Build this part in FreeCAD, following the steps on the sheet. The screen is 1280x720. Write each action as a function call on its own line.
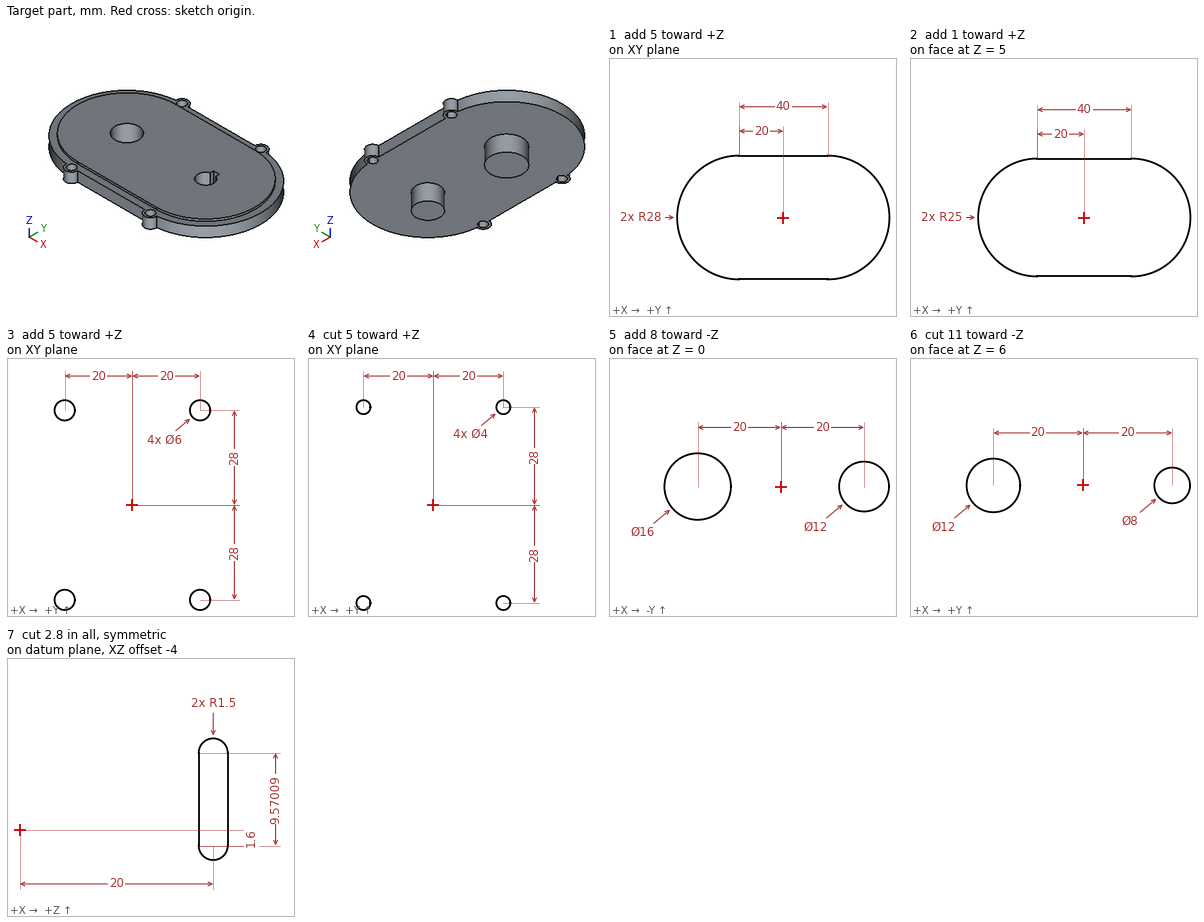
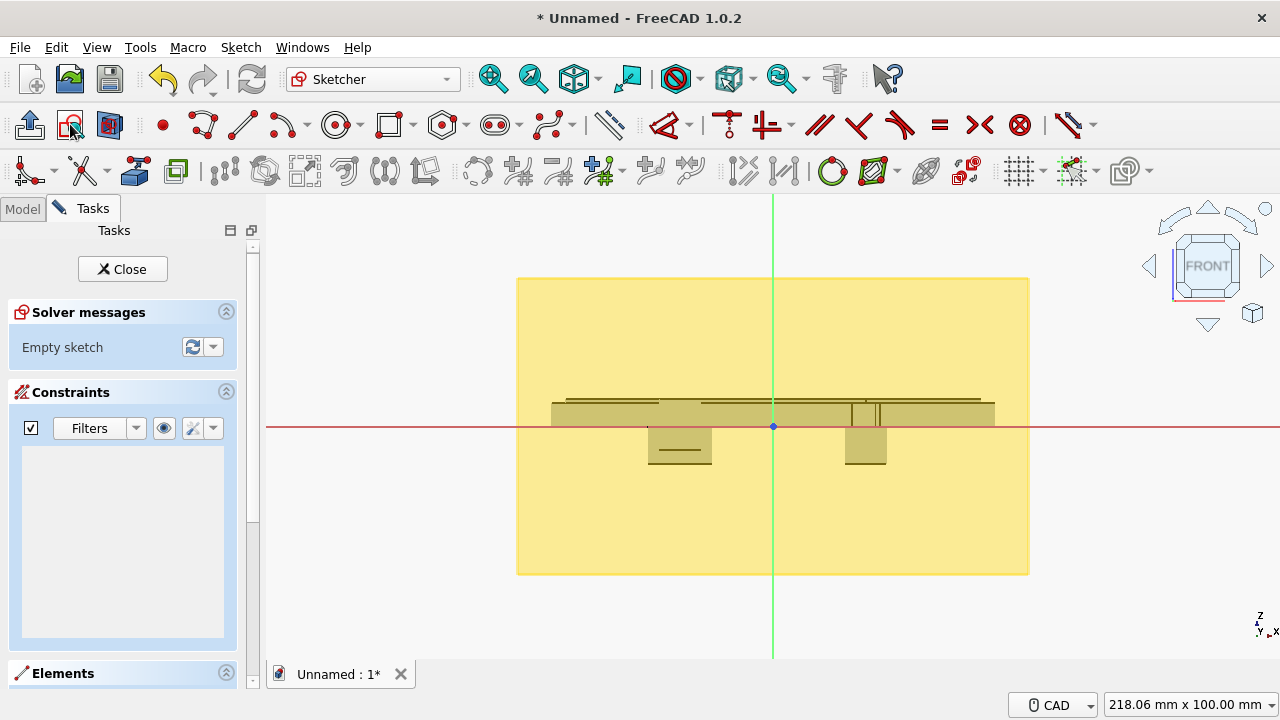
scroll(853, 408, up, 8)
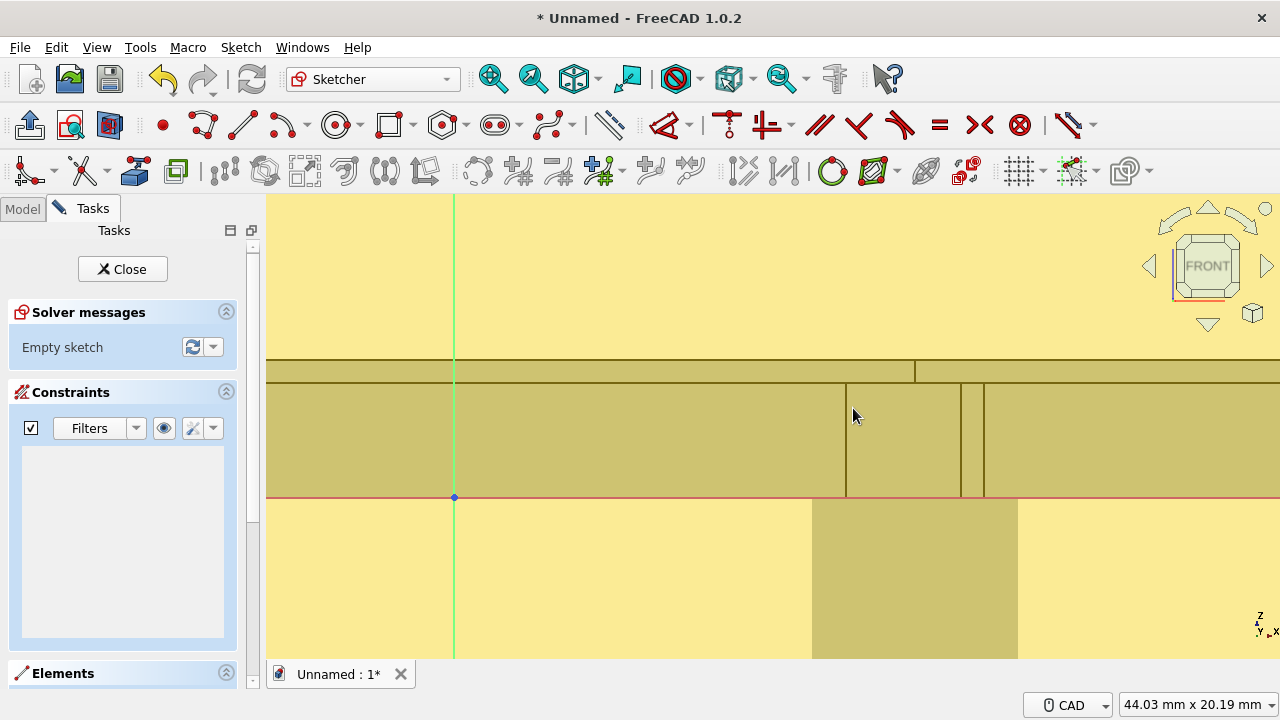
click(496, 126)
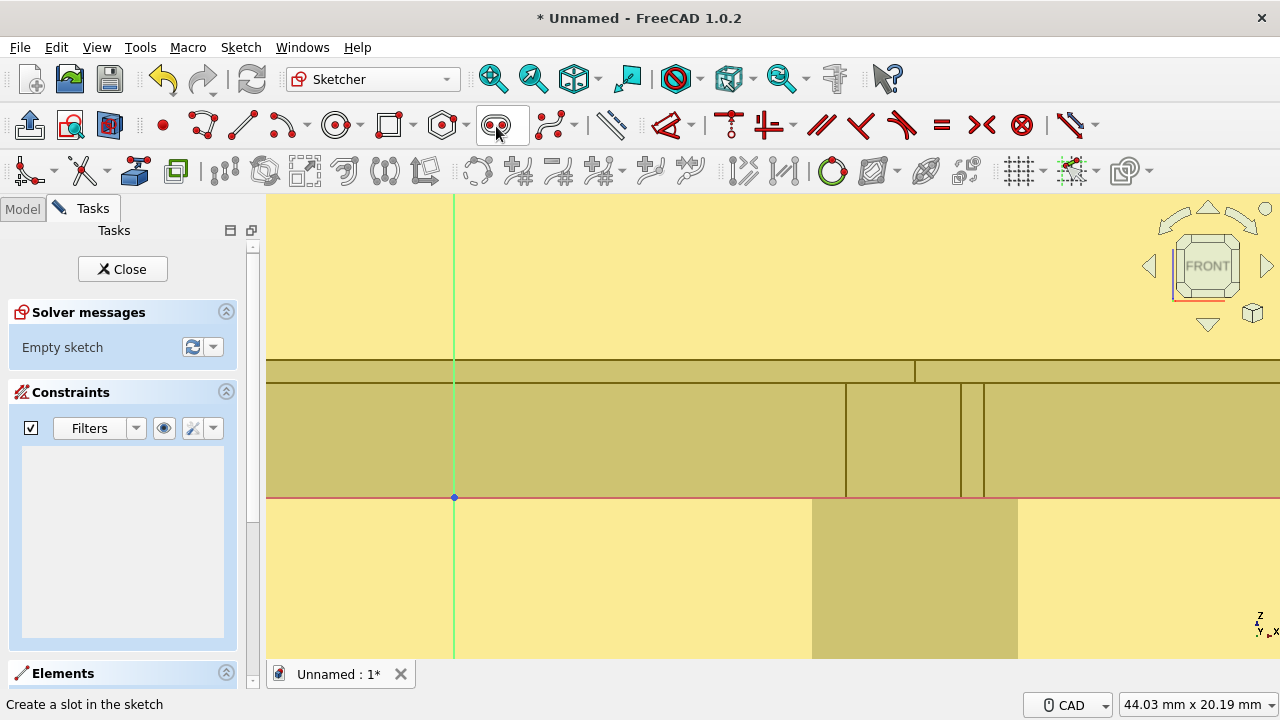
click(915, 535)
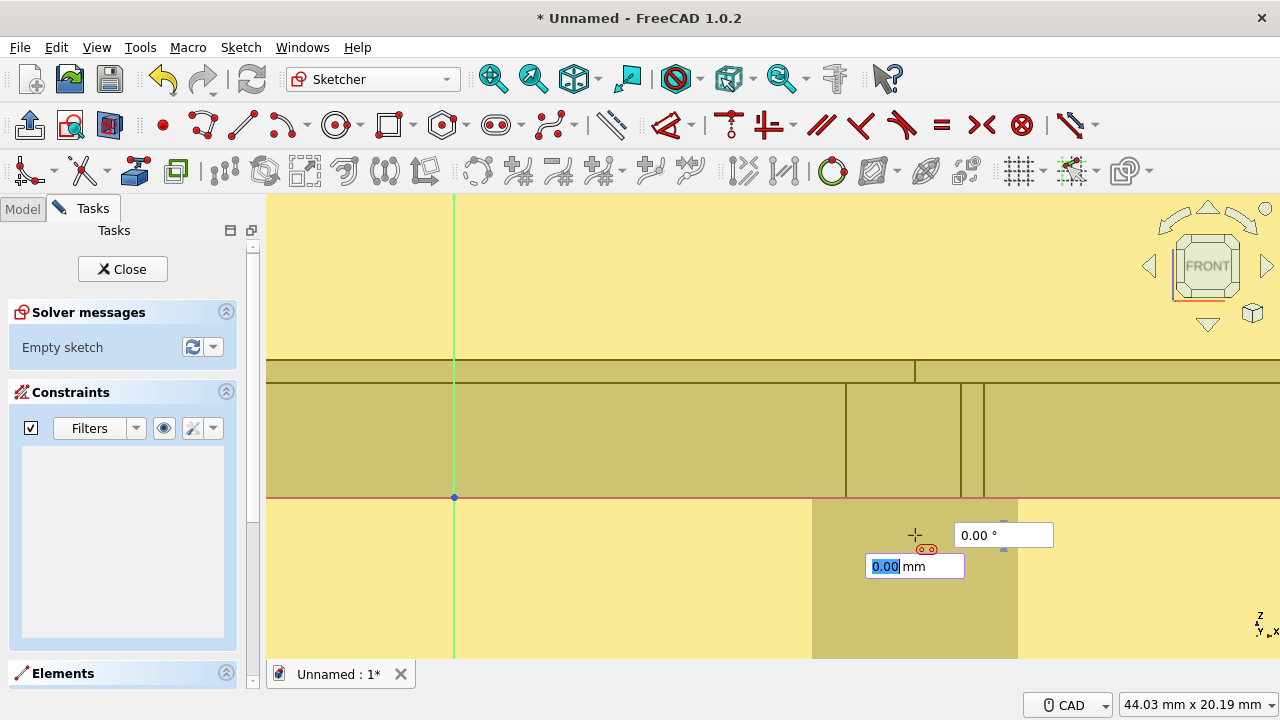
click(915, 314)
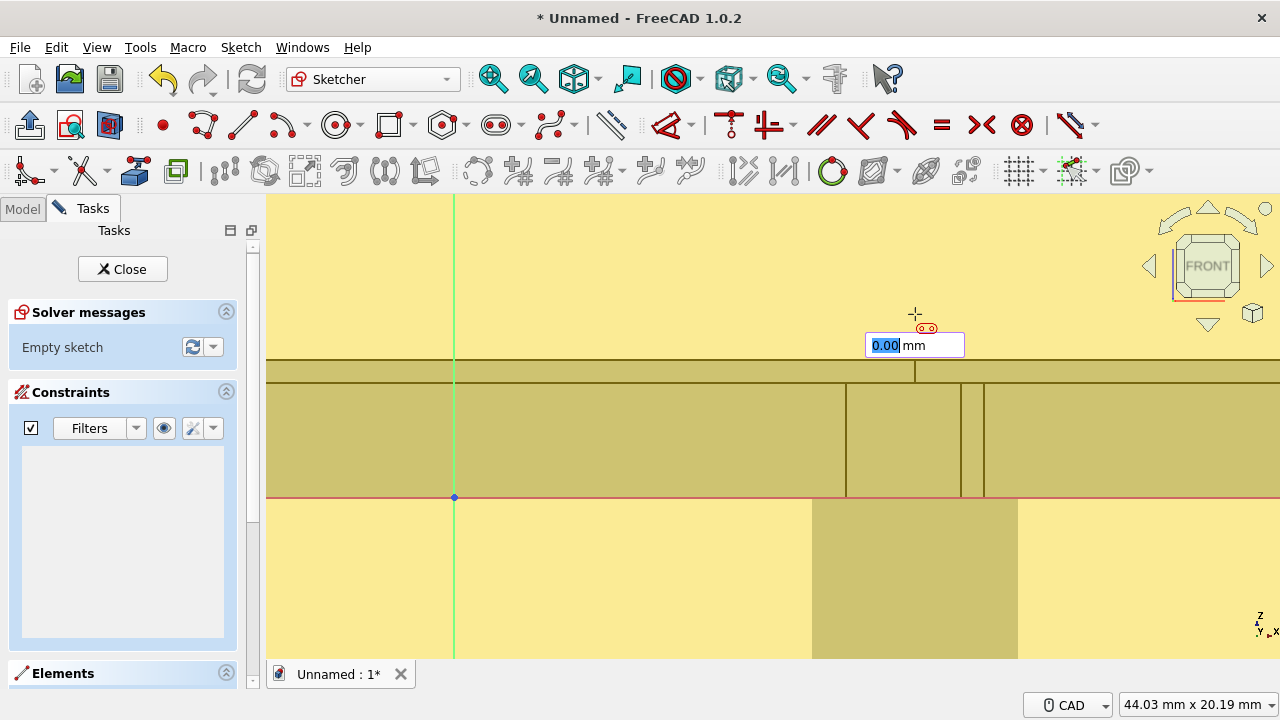
click(881, 424)
key(Escape)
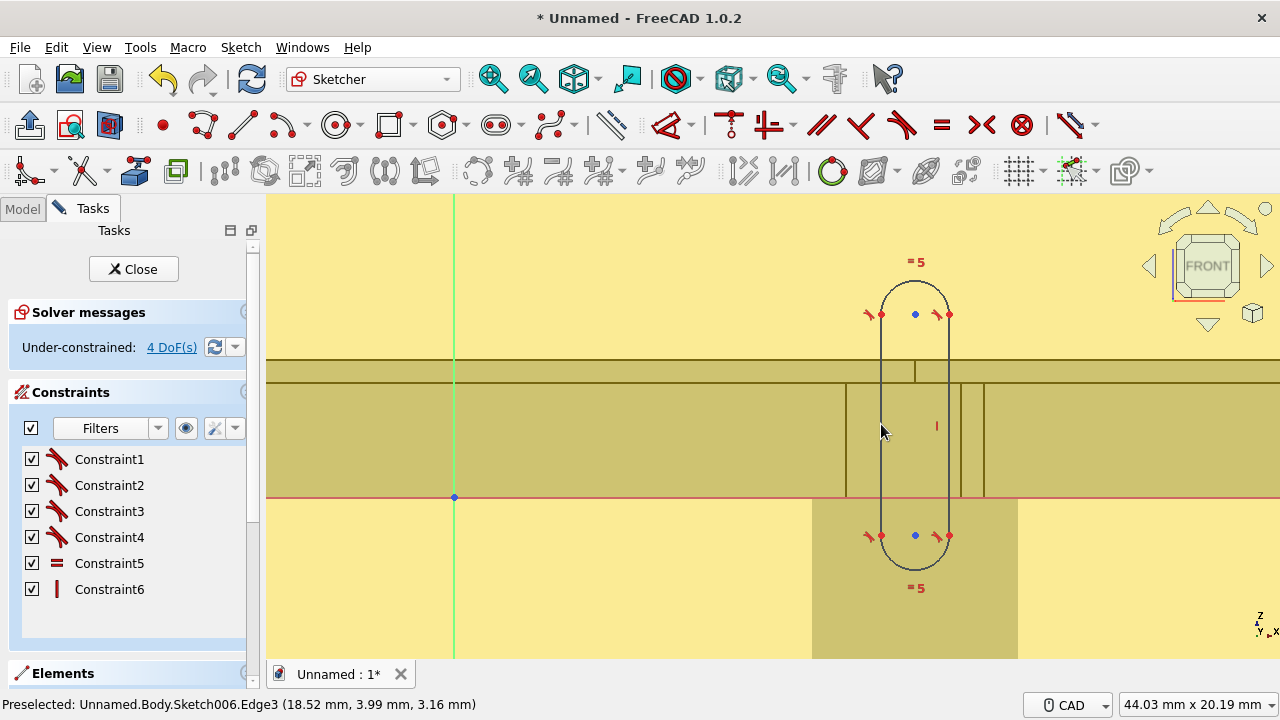
key(d)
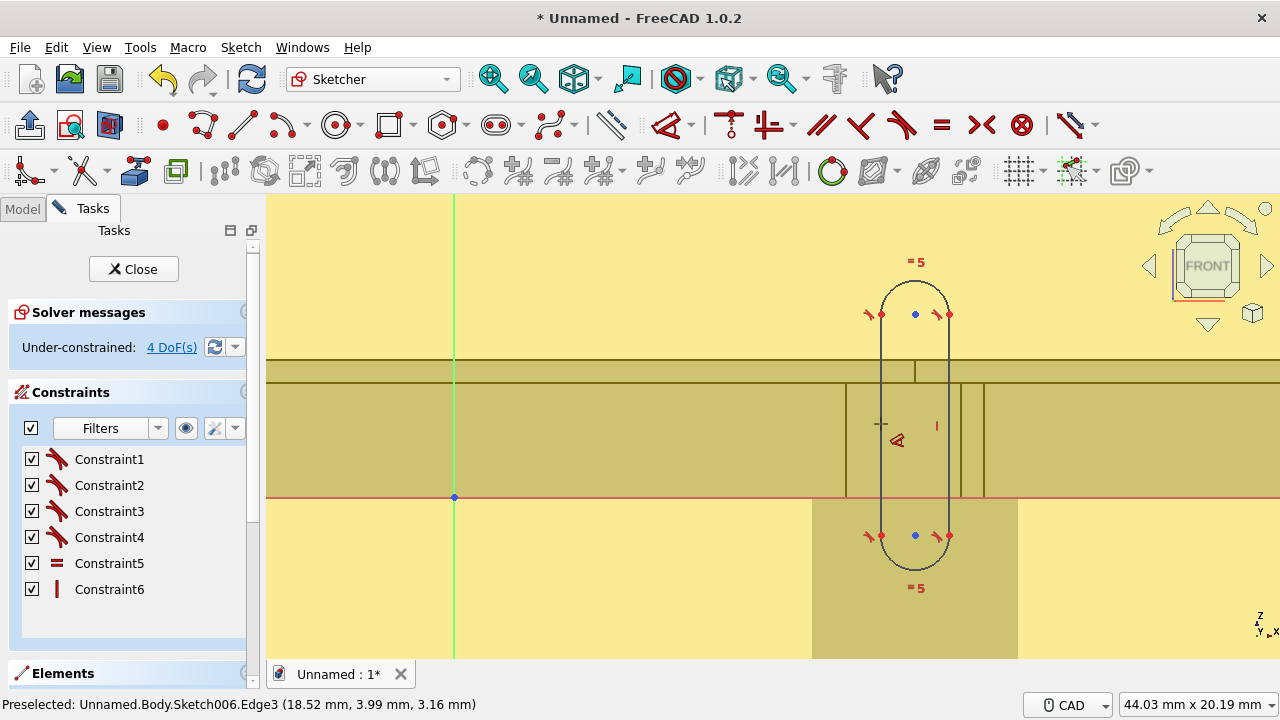
click(895, 564)
click(876, 590)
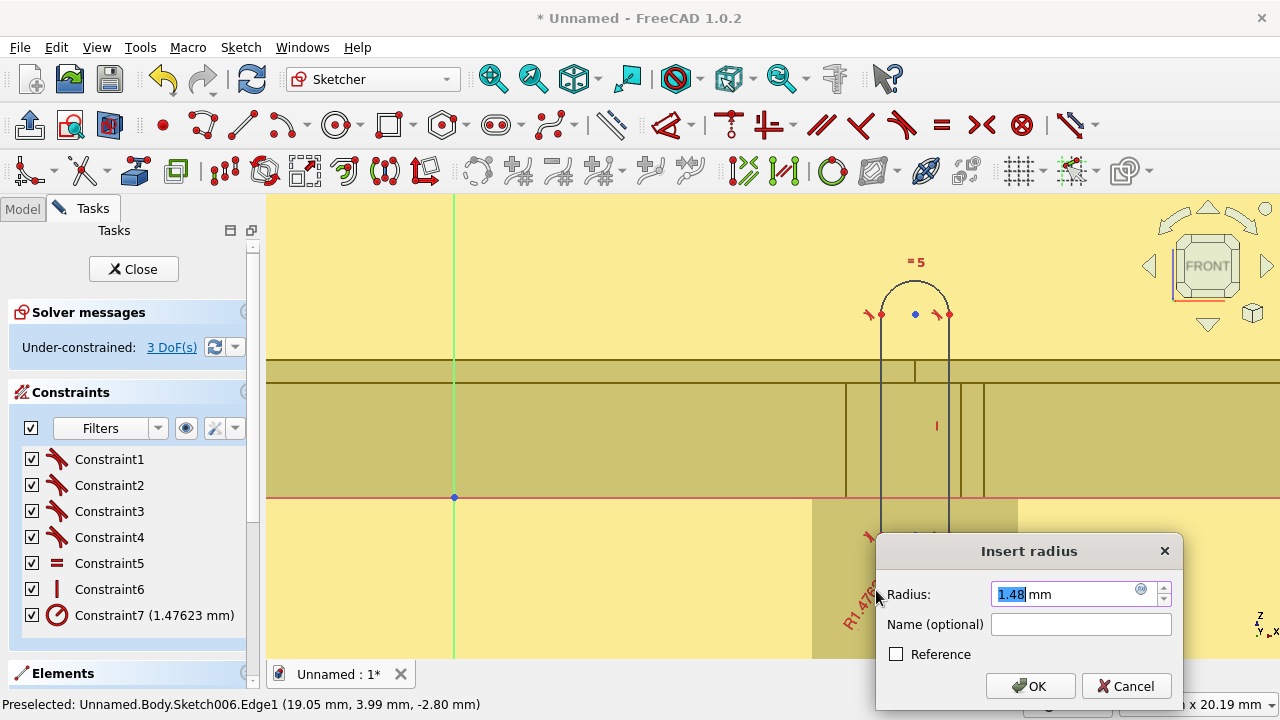
text(1.5)
key(Return)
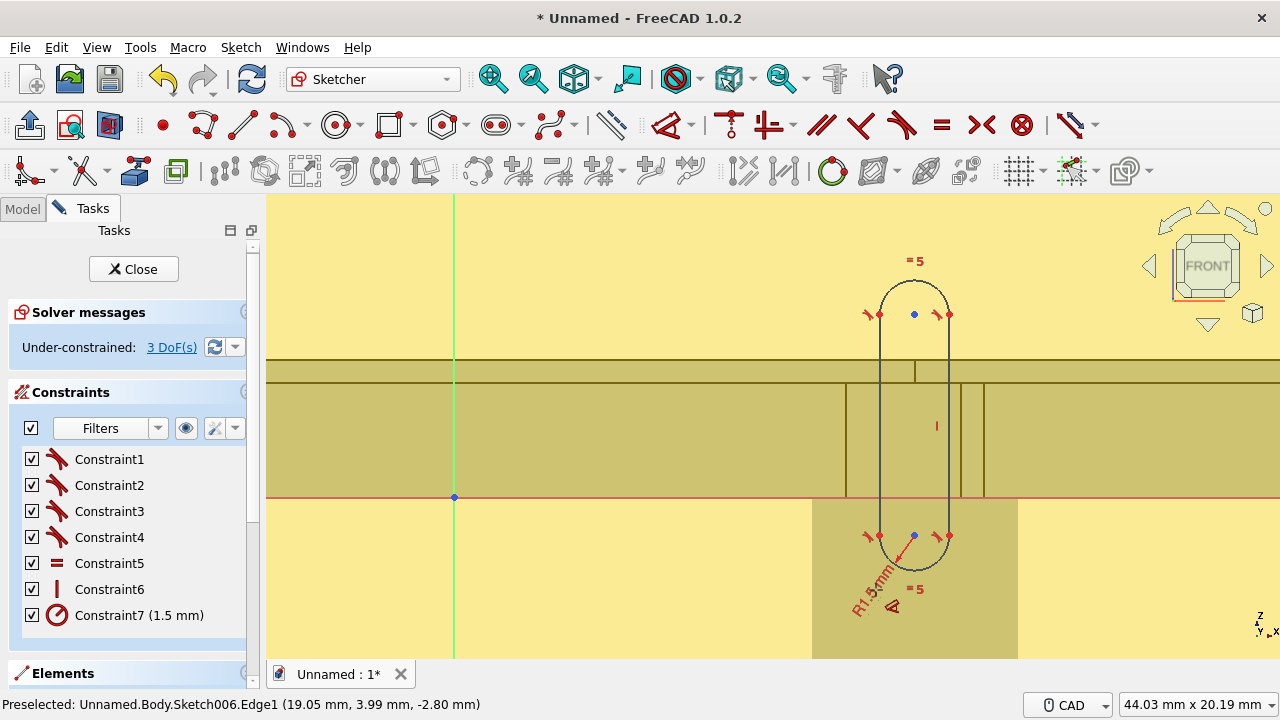
click(914, 536)
click(684, 570)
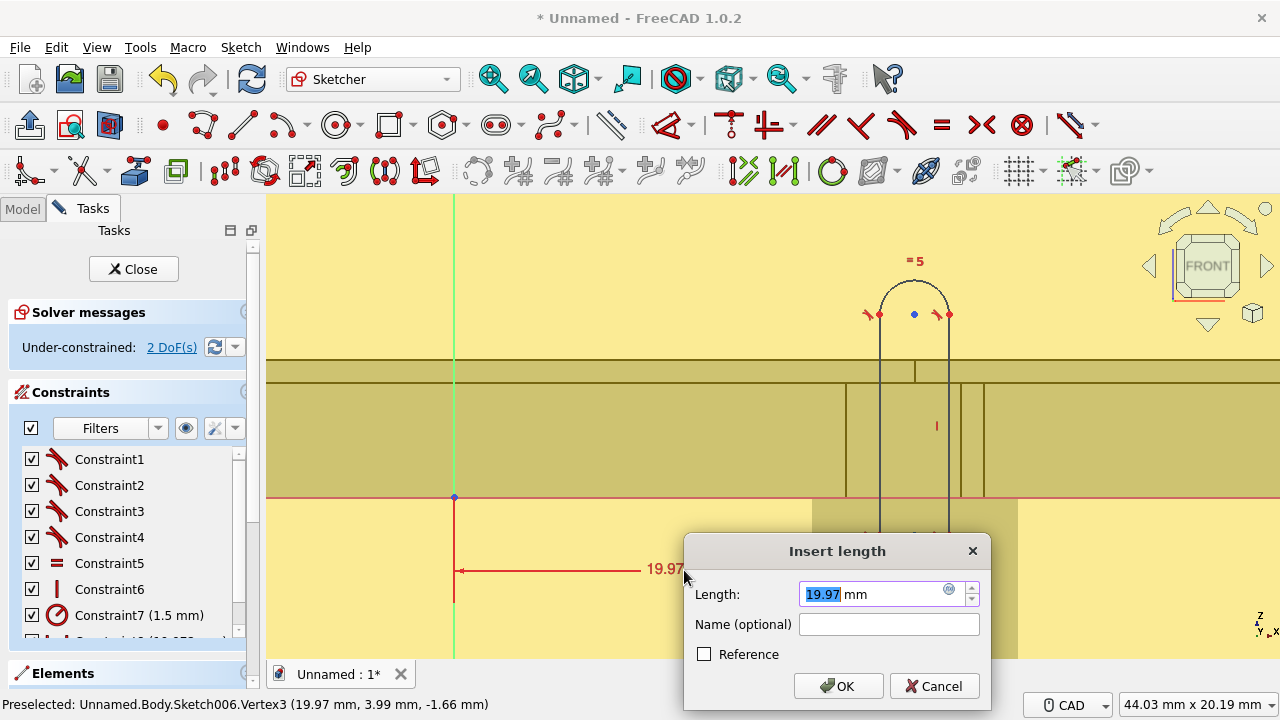
text(20)
key(Return)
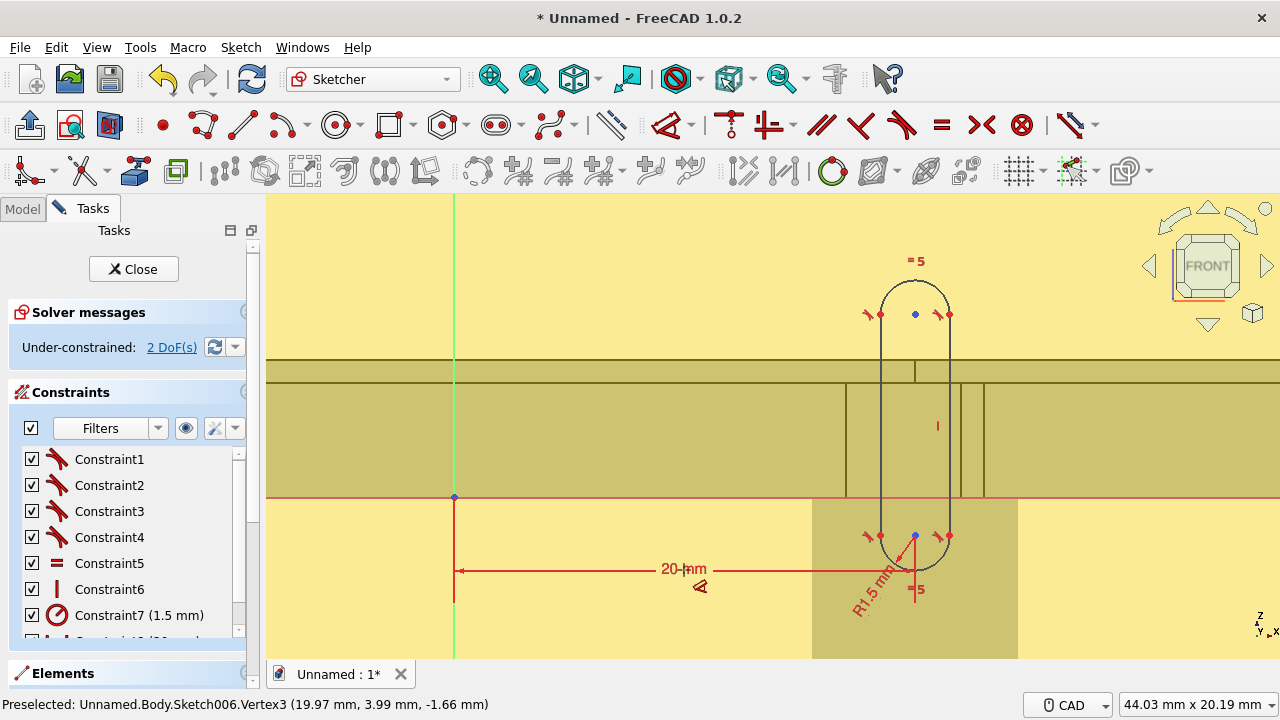
click(881, 536)
click(420, 517)